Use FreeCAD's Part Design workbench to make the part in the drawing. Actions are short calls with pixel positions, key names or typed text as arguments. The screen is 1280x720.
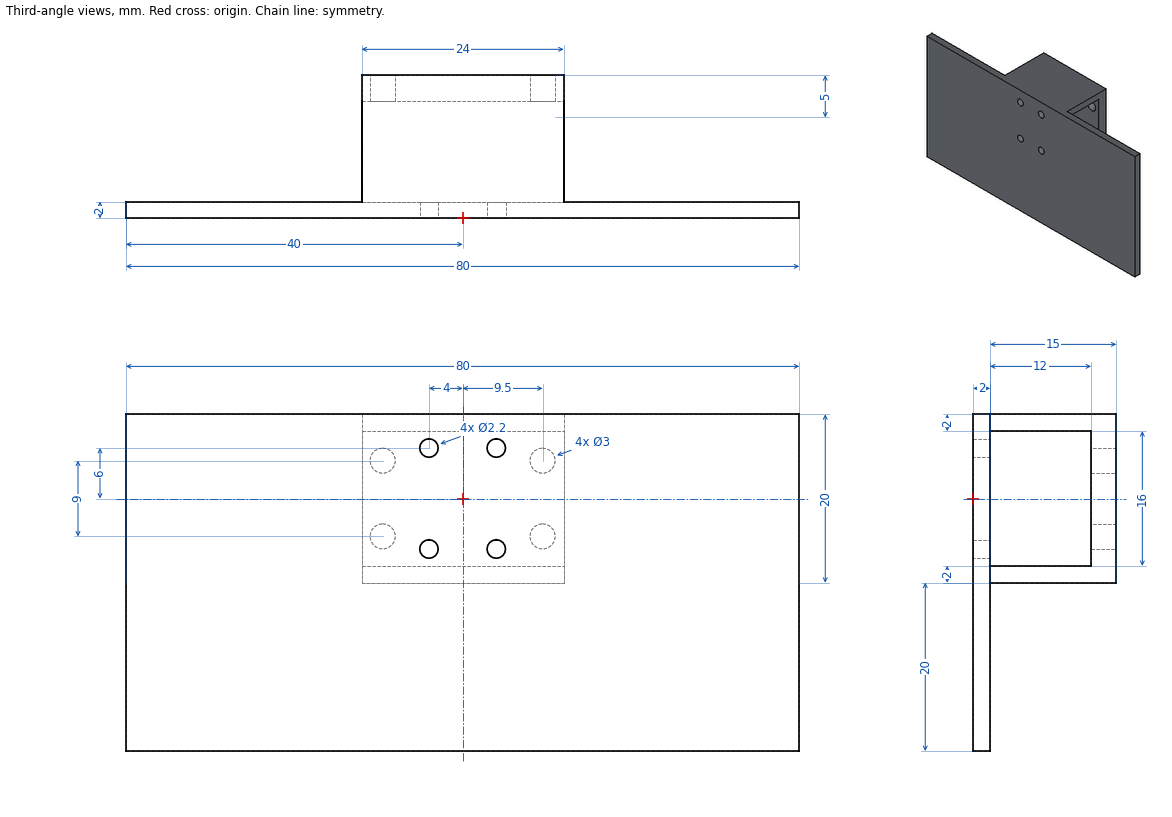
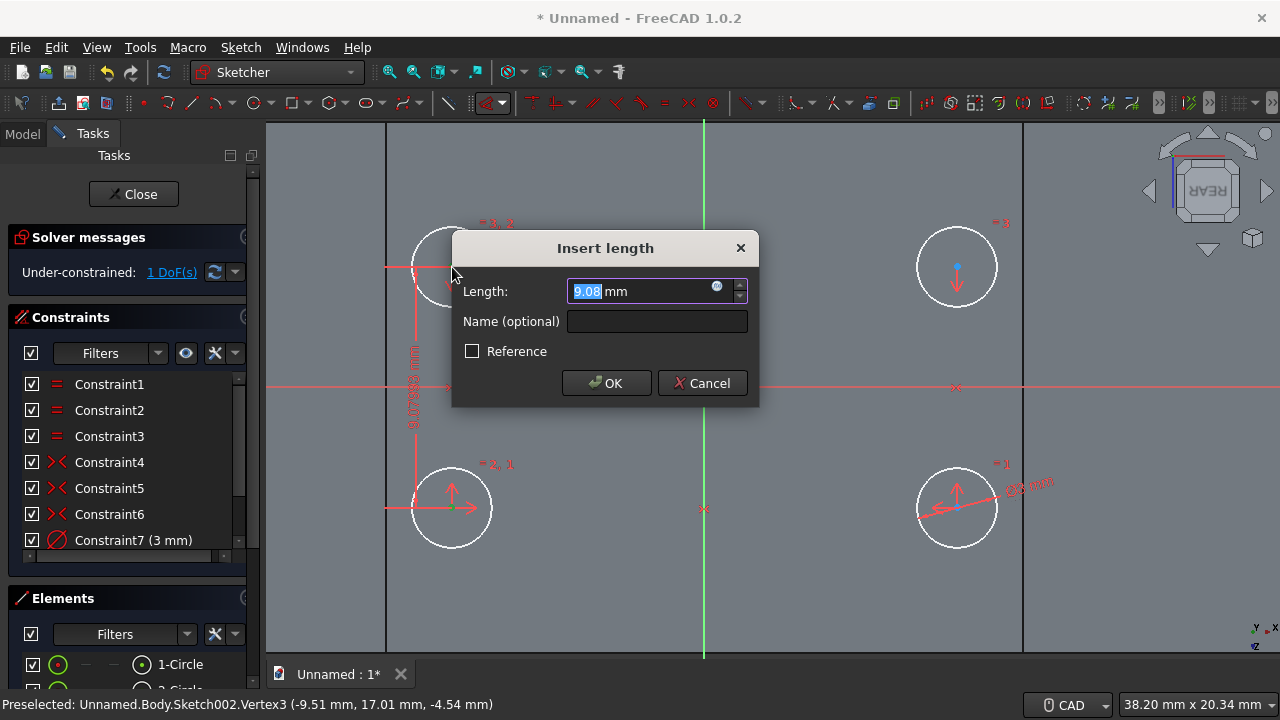
text(9)
key(Return)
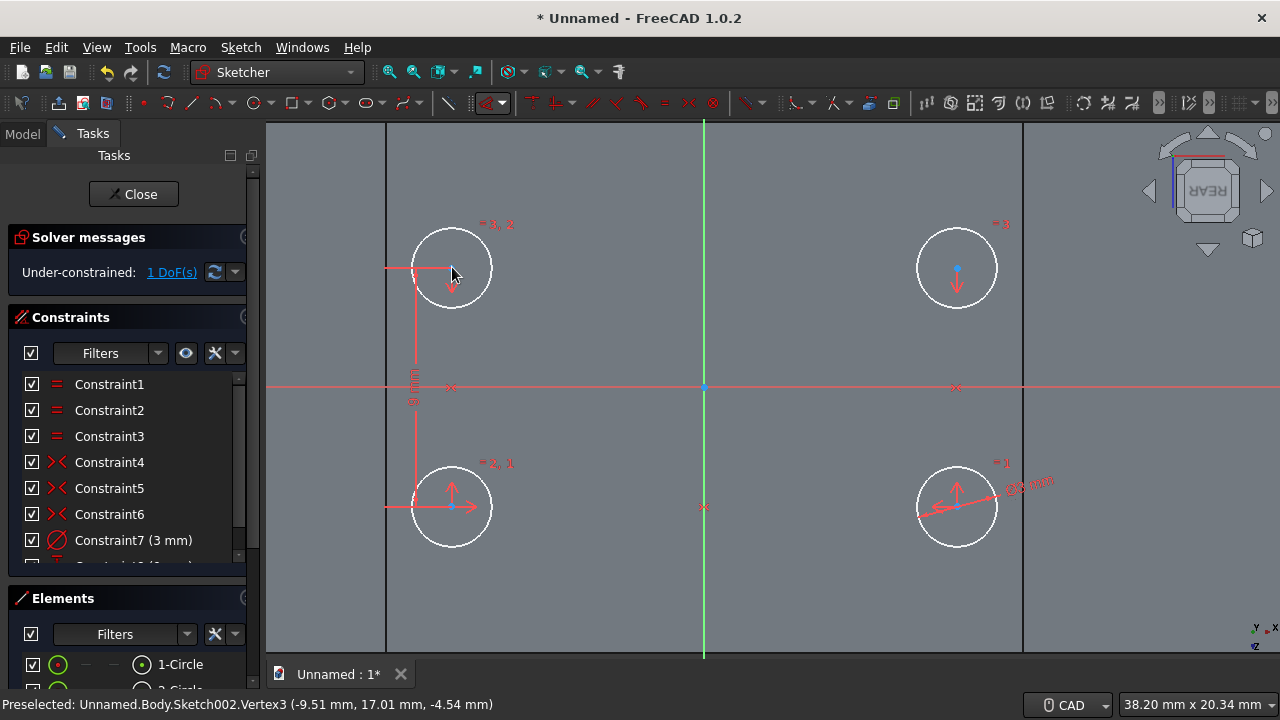
click(957, 507)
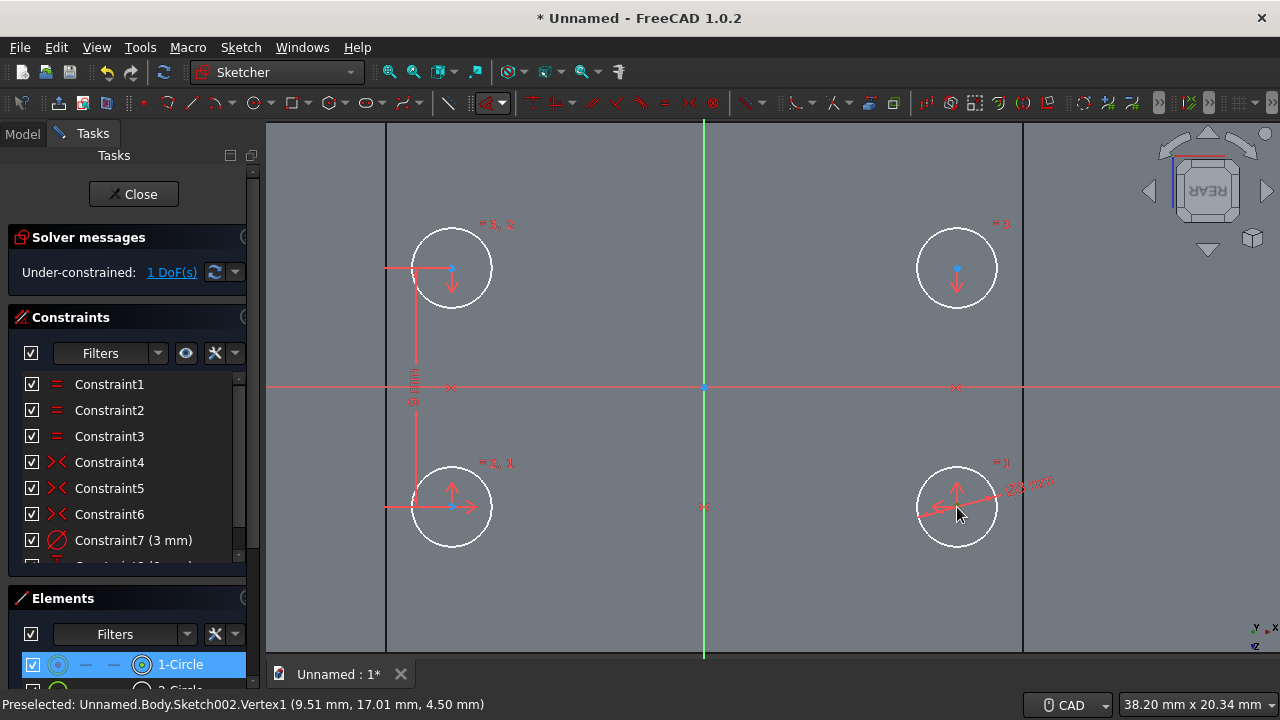
click(504, 104)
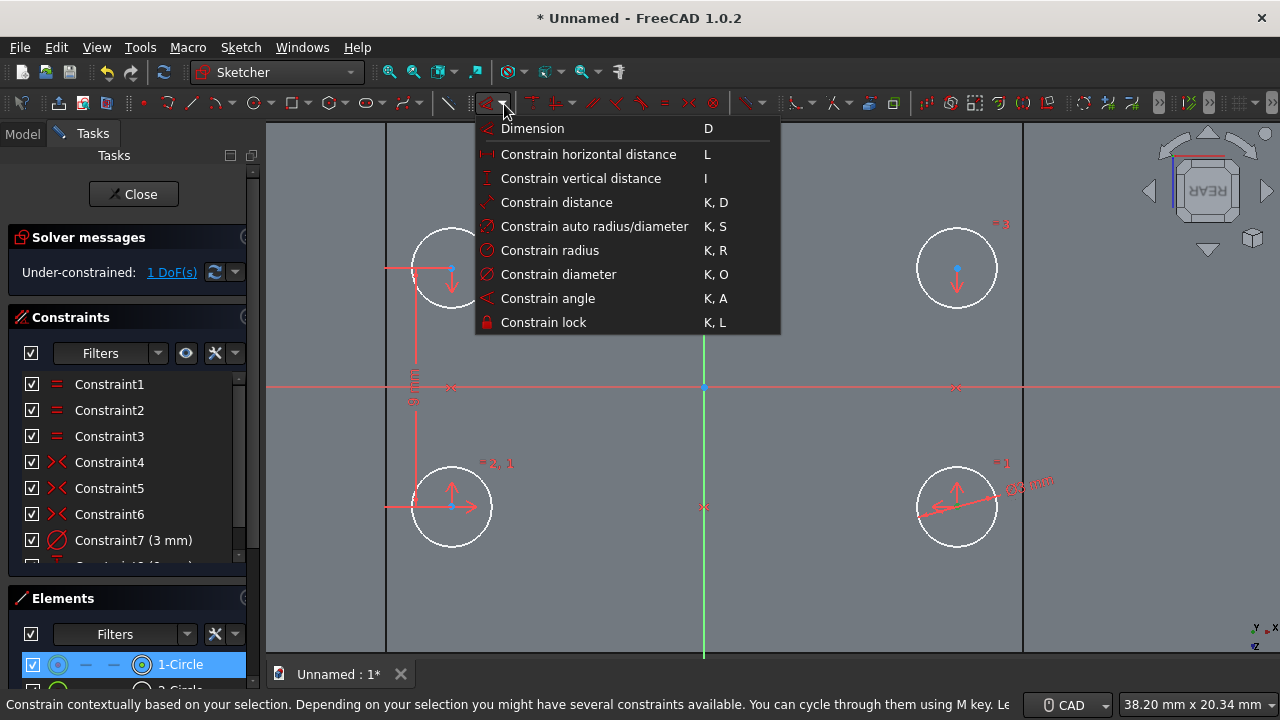
click(628, 154)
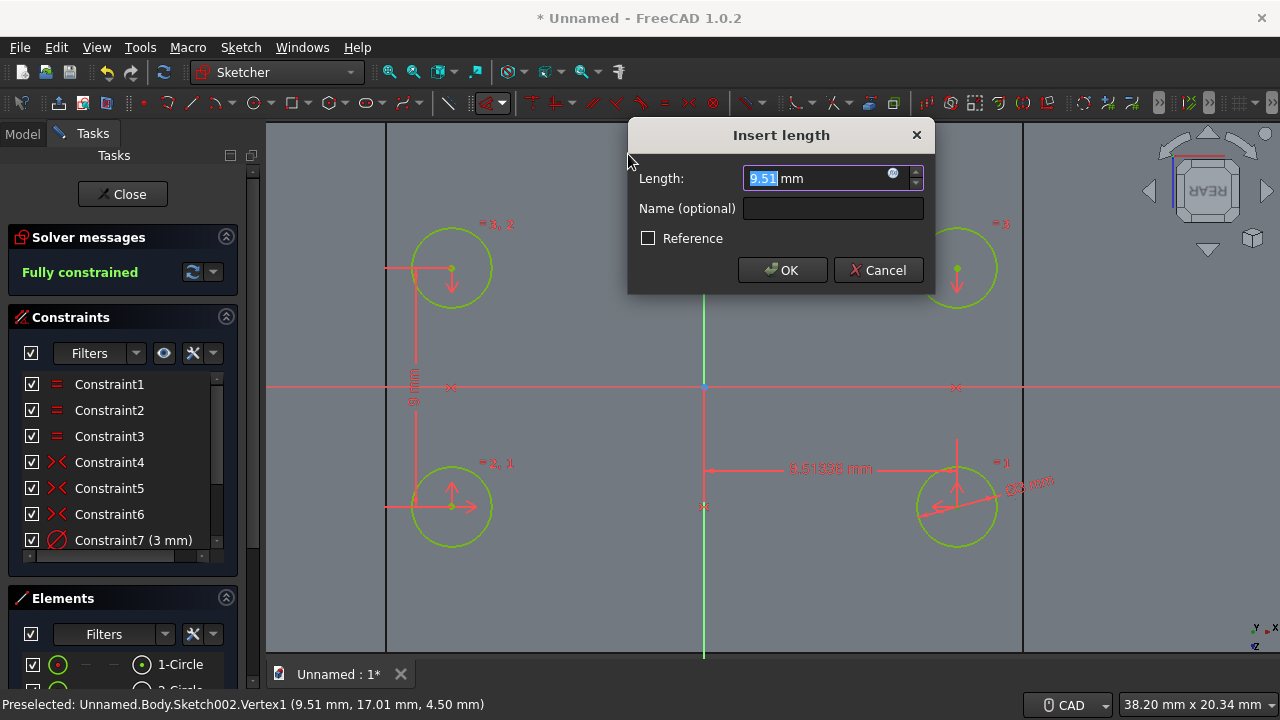
text(9.5)
key(Return)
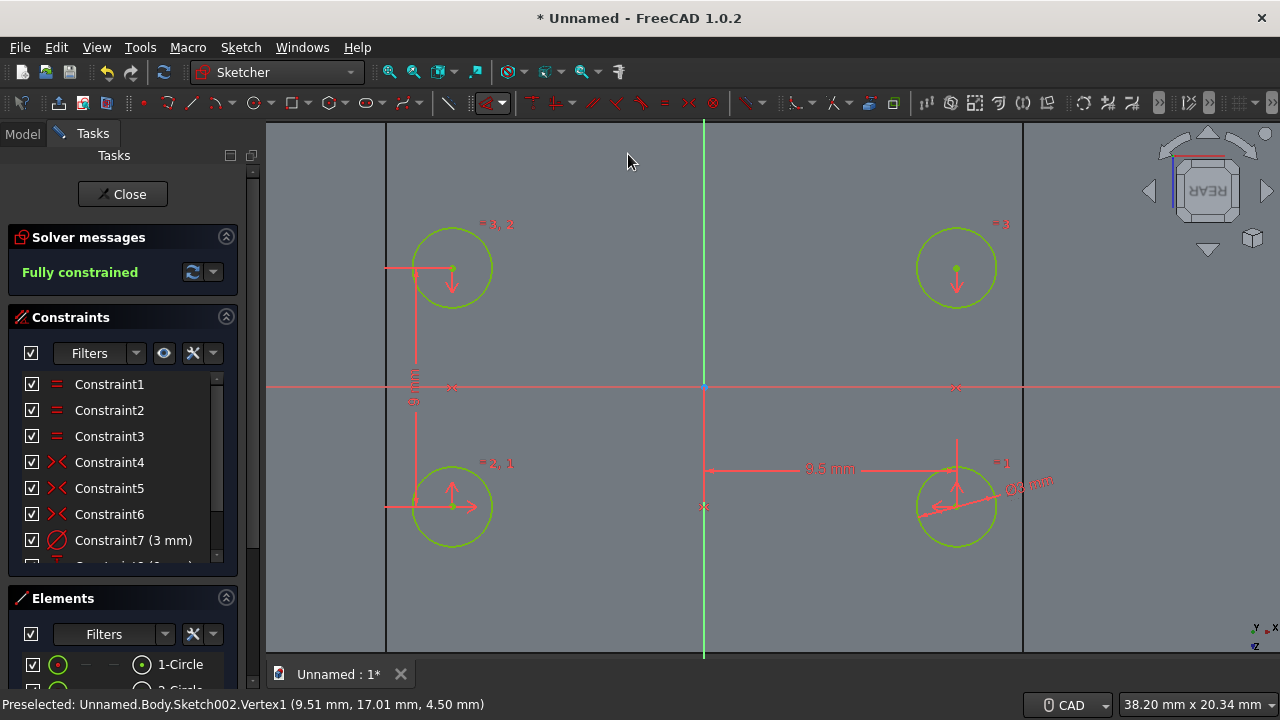
click(123, 194)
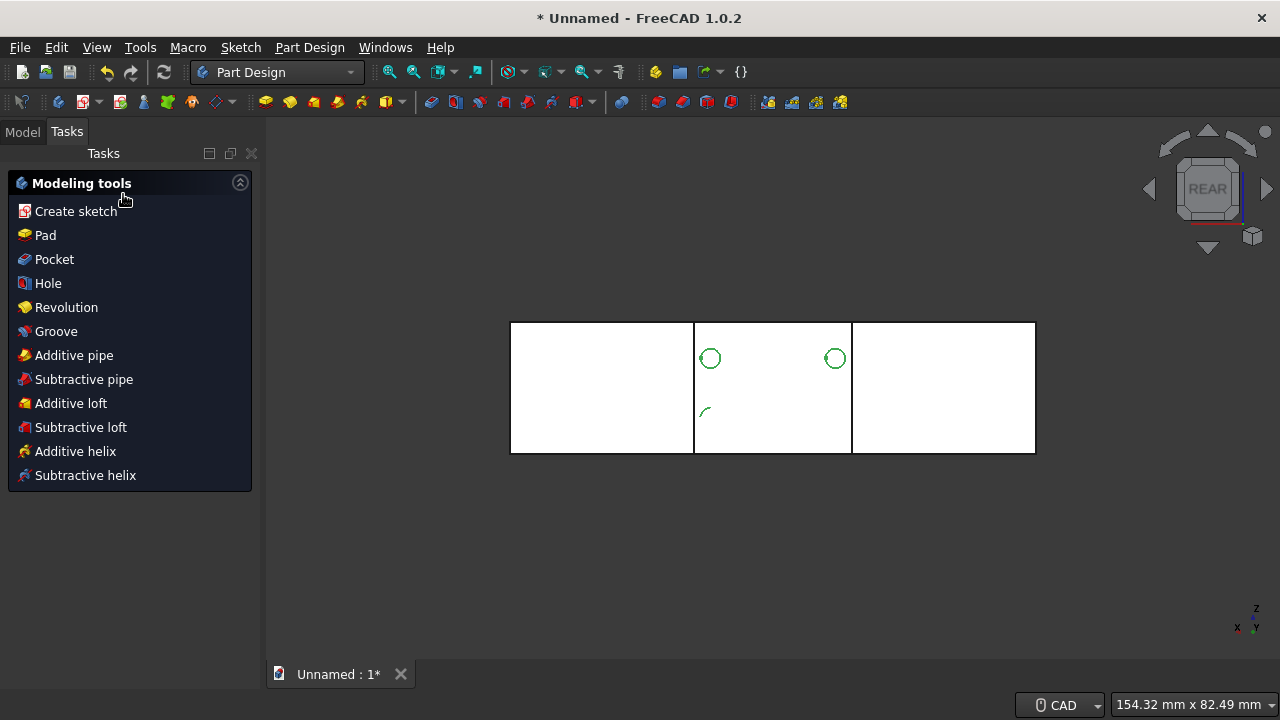
click(432, 102)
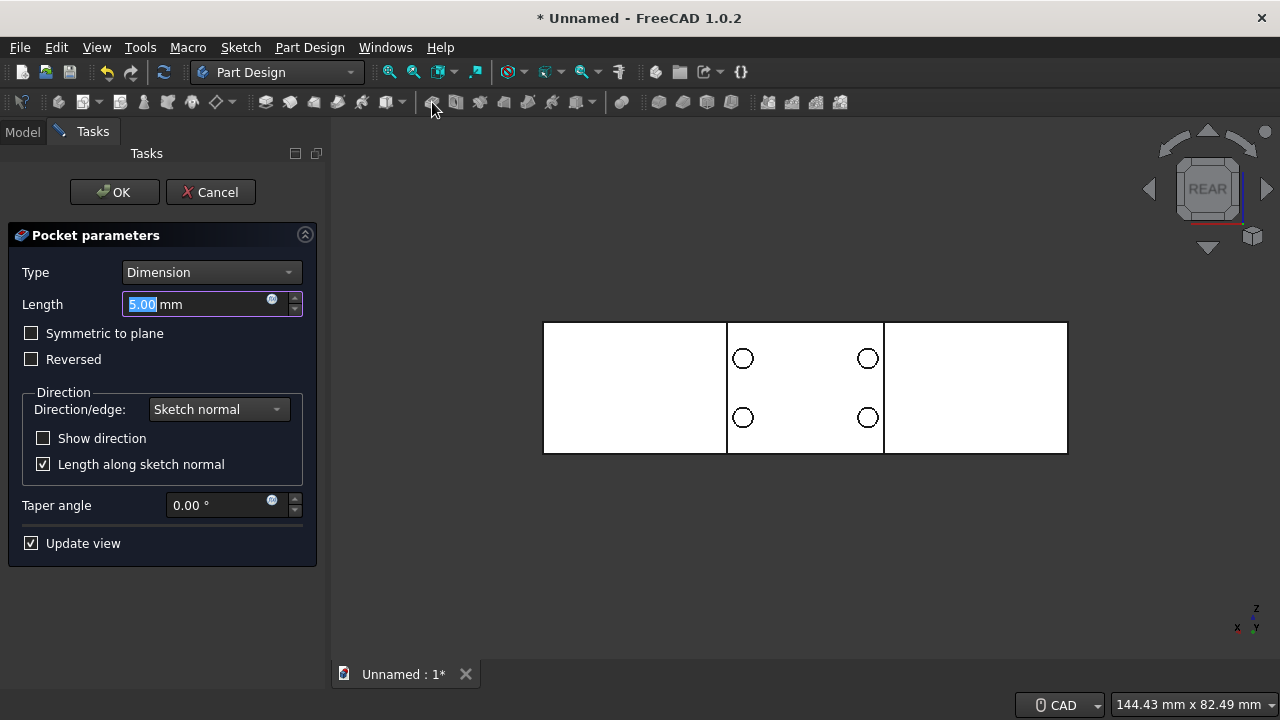
text(5)
key(Tab)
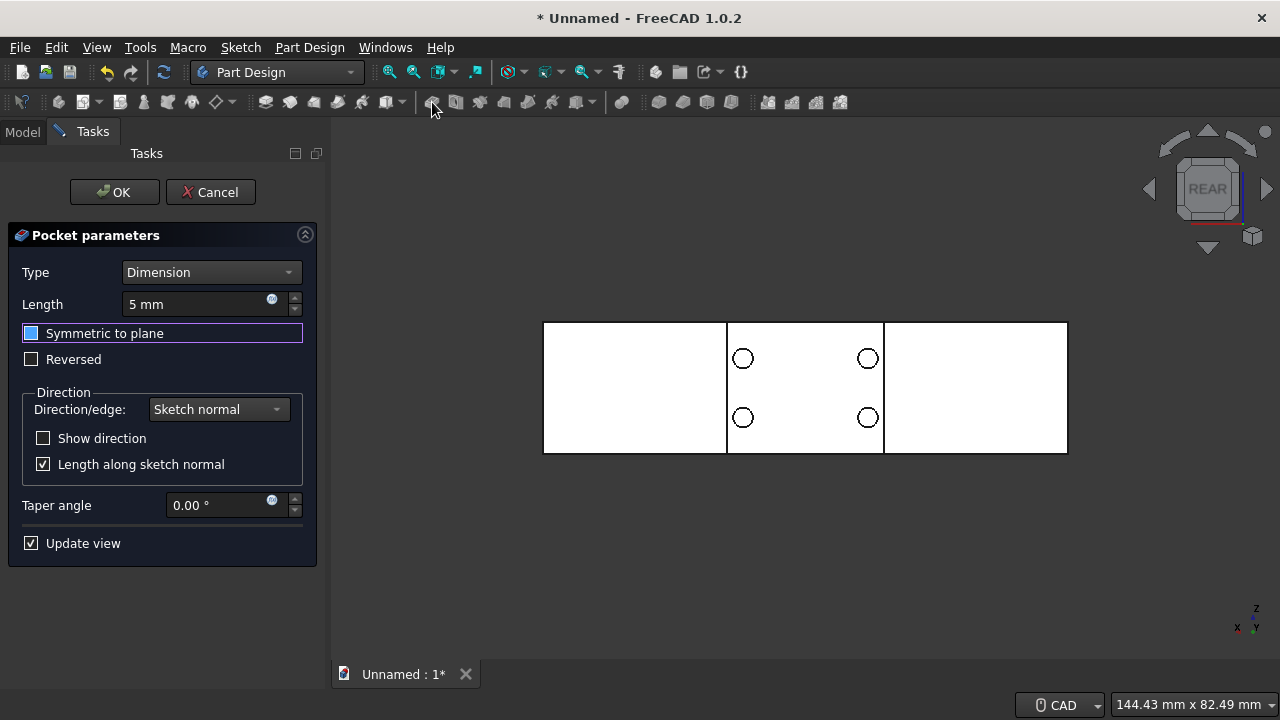
click(115, 192)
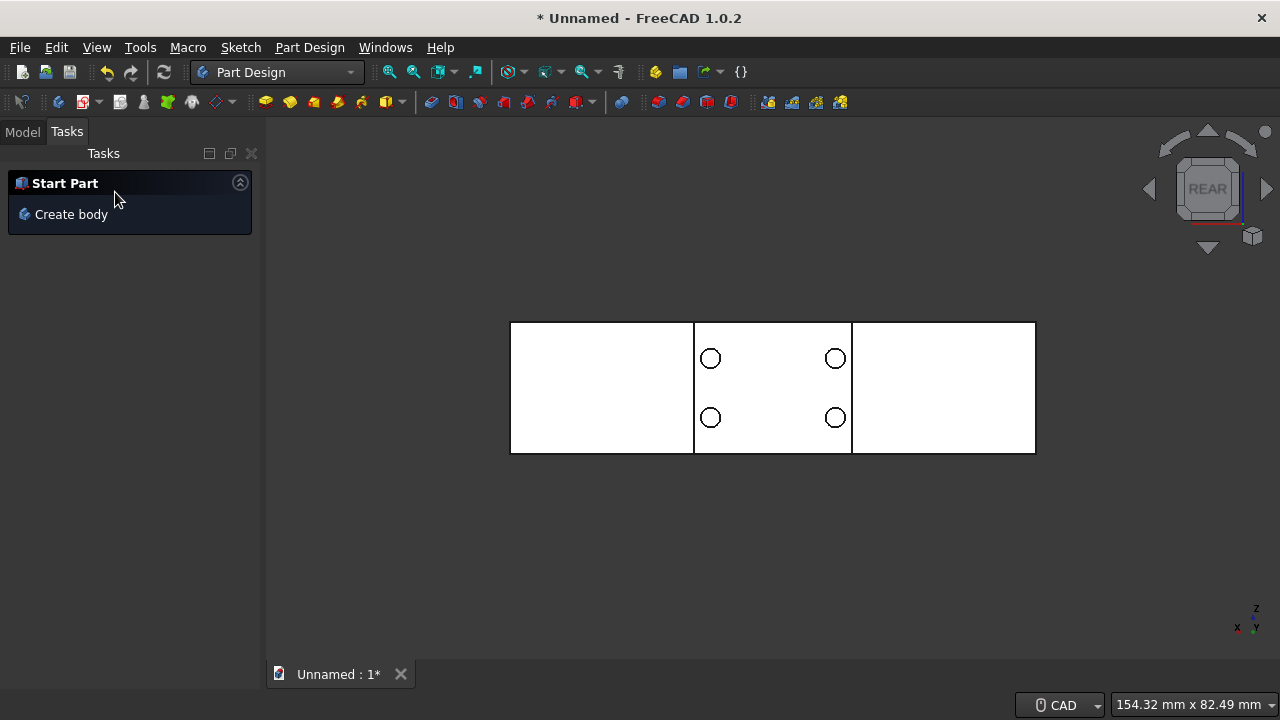
key(5)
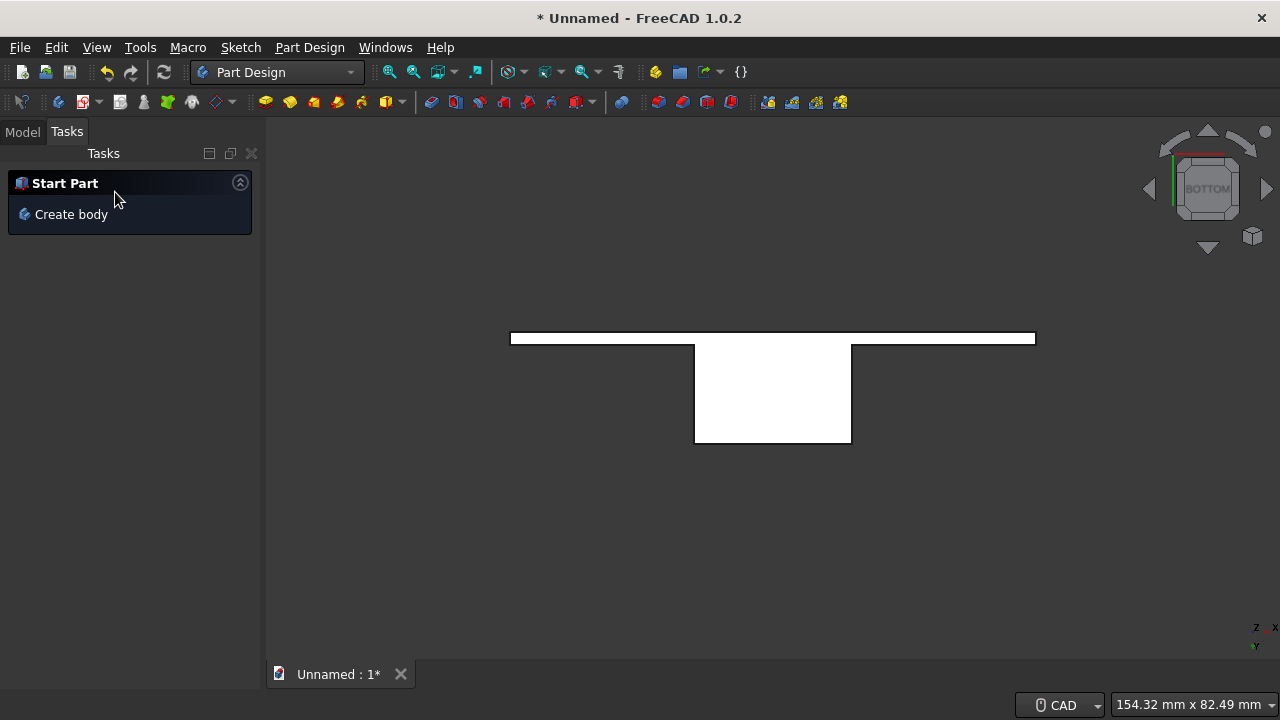
click(773, 387)